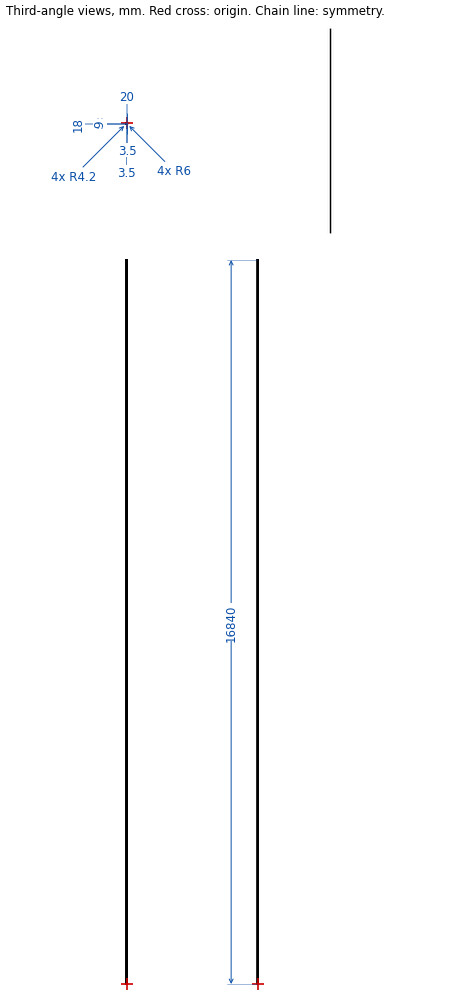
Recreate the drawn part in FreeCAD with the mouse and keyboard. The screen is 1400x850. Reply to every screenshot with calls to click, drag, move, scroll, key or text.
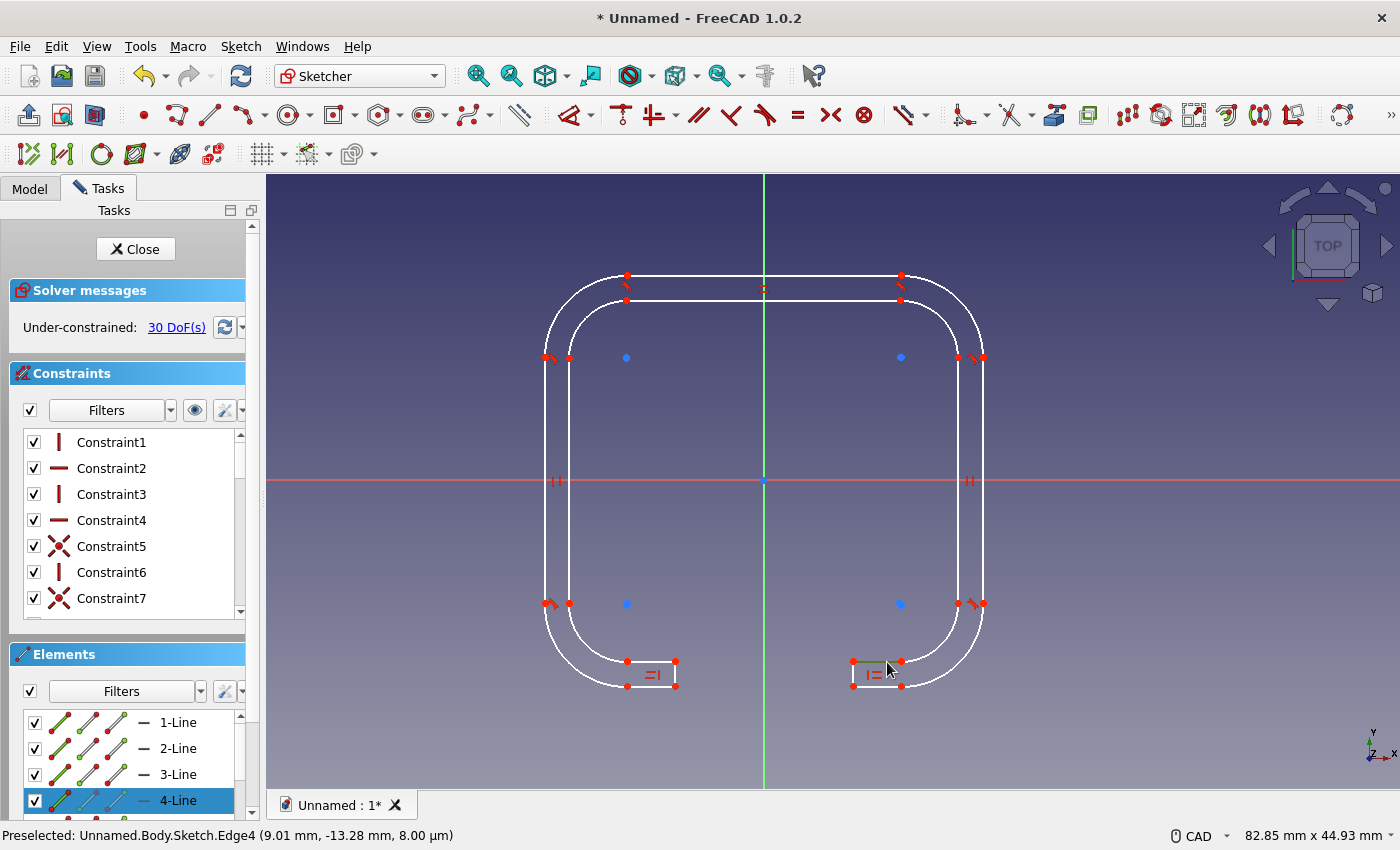
click(927, 655)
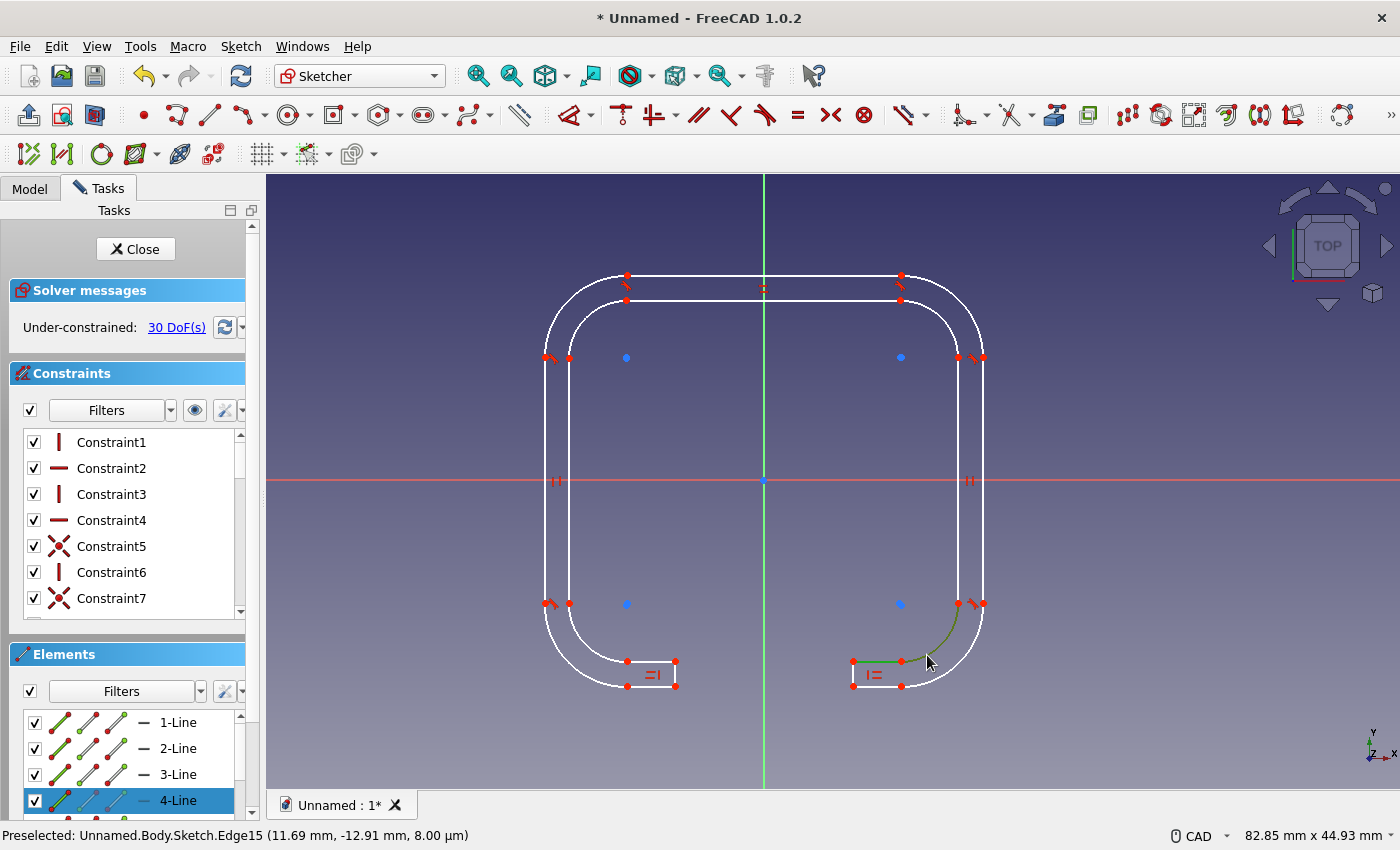
click(765, 116)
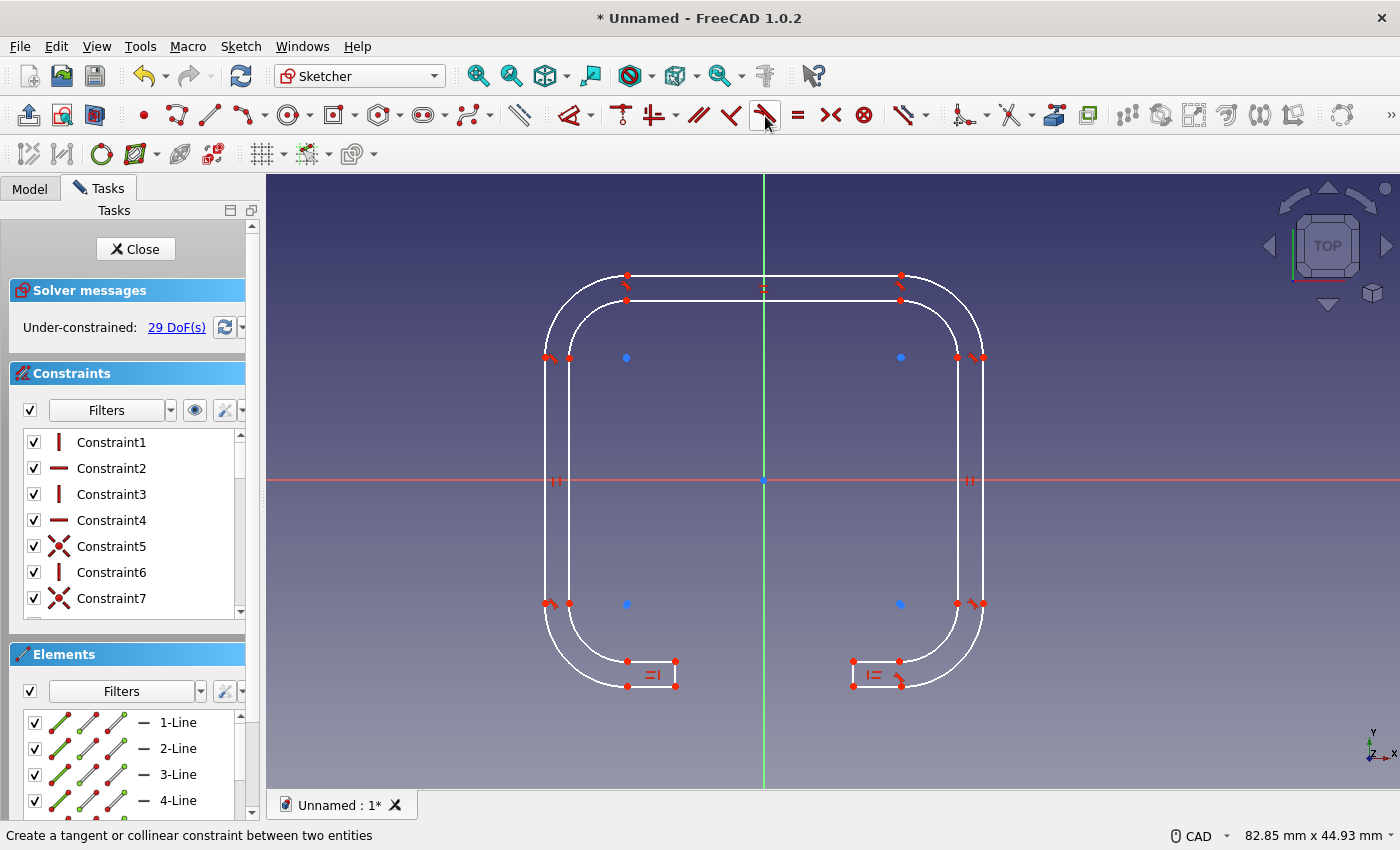
click(867, 687)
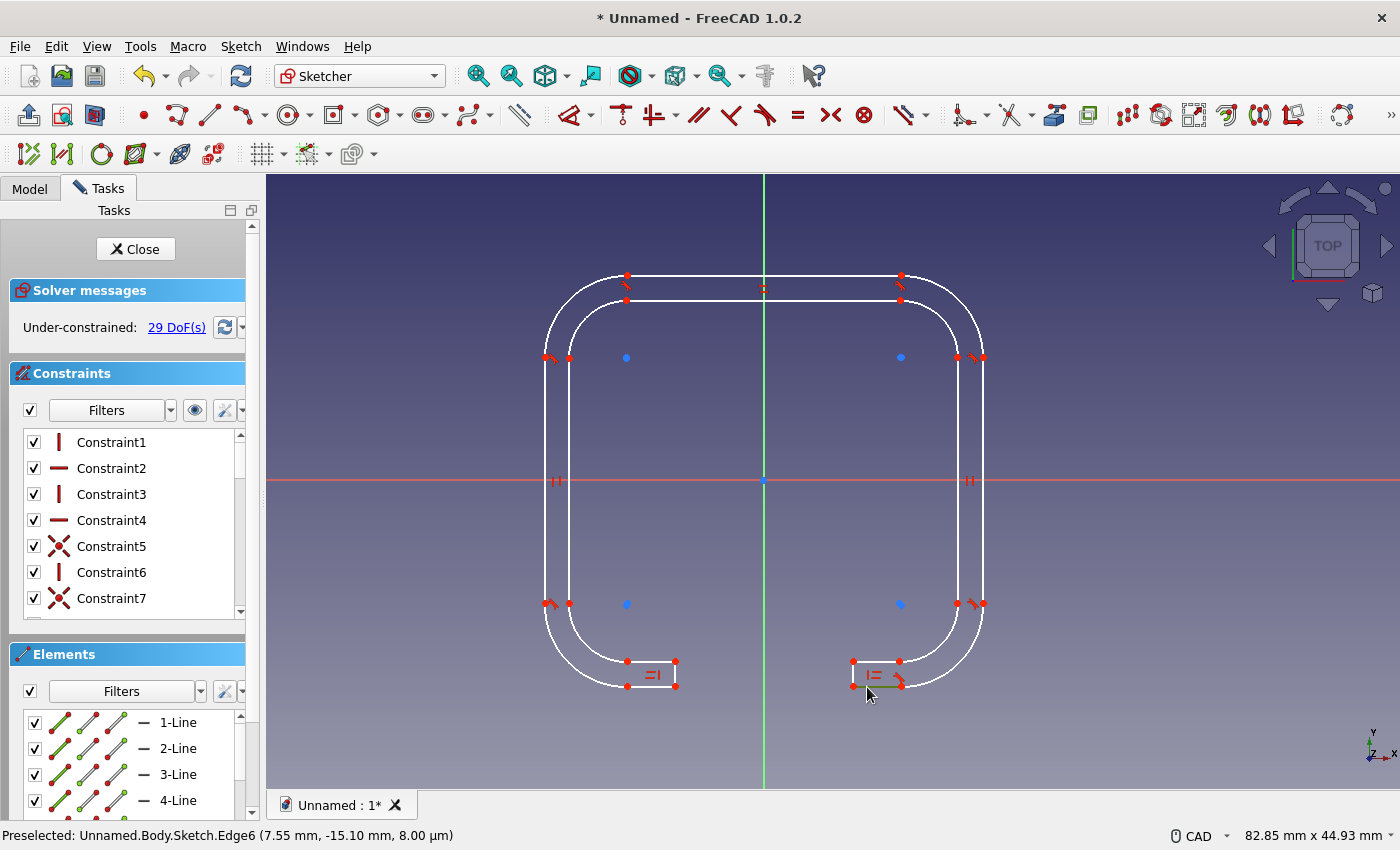
click(939, 678)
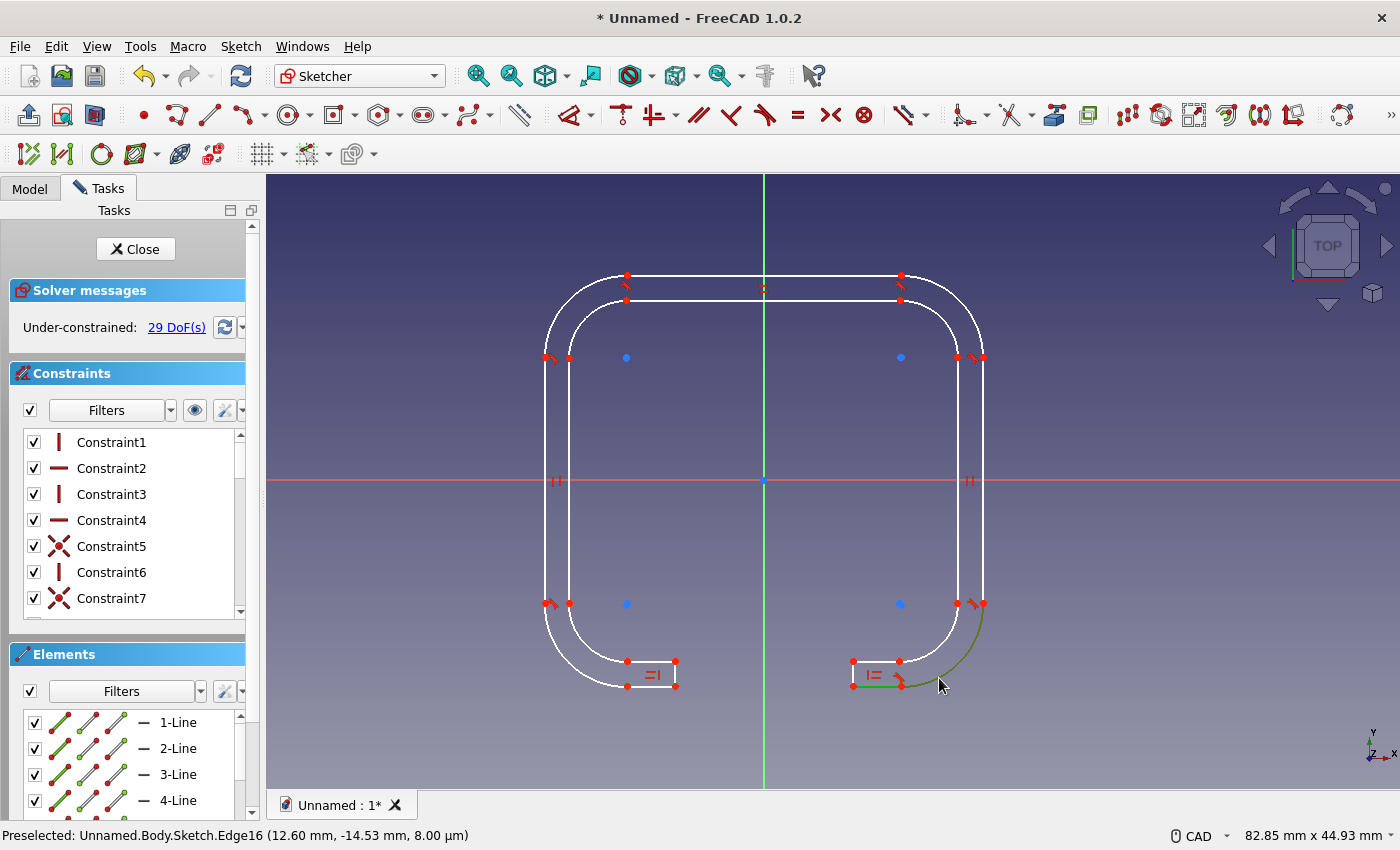
click(765, 116)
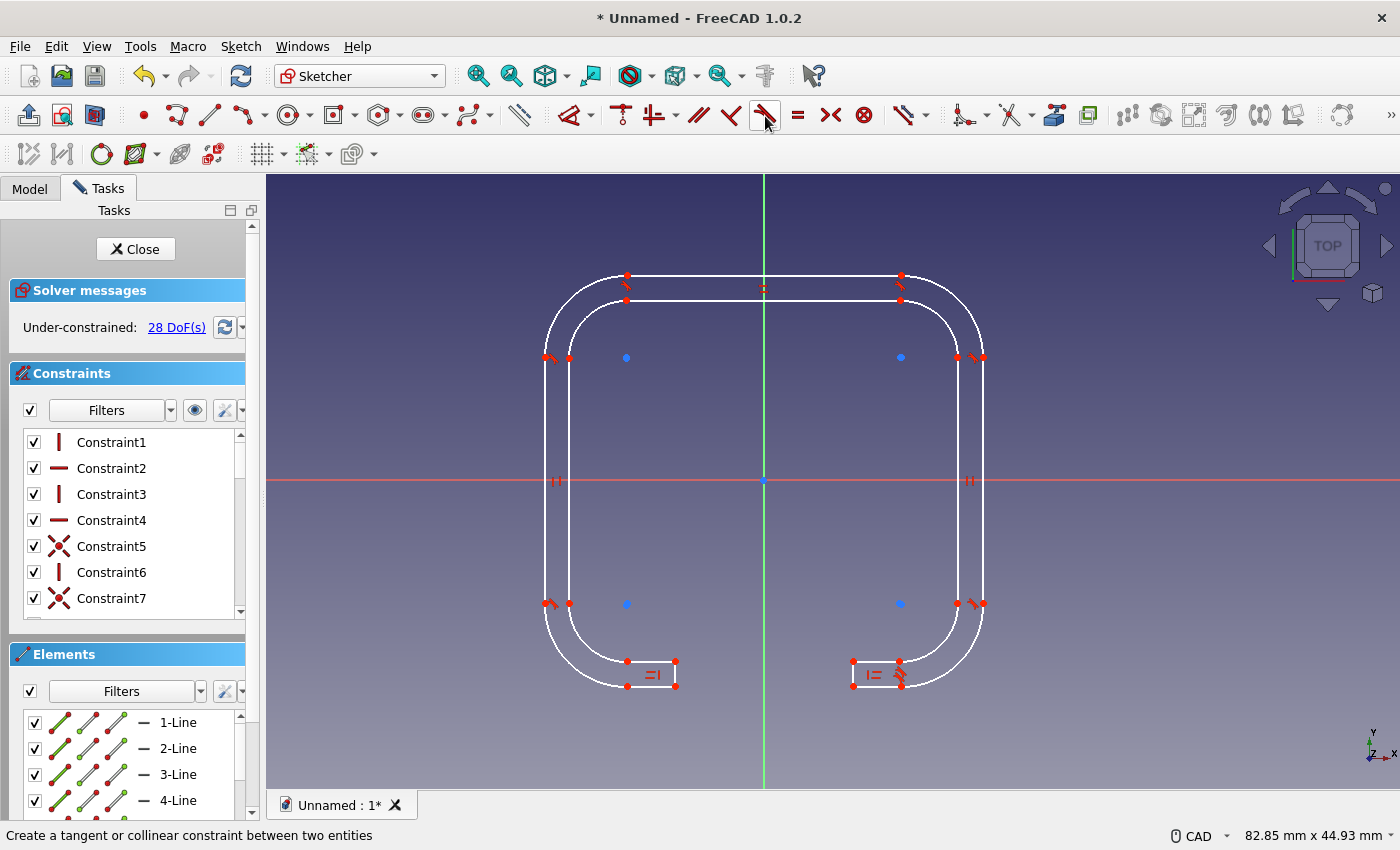
click(983, 530)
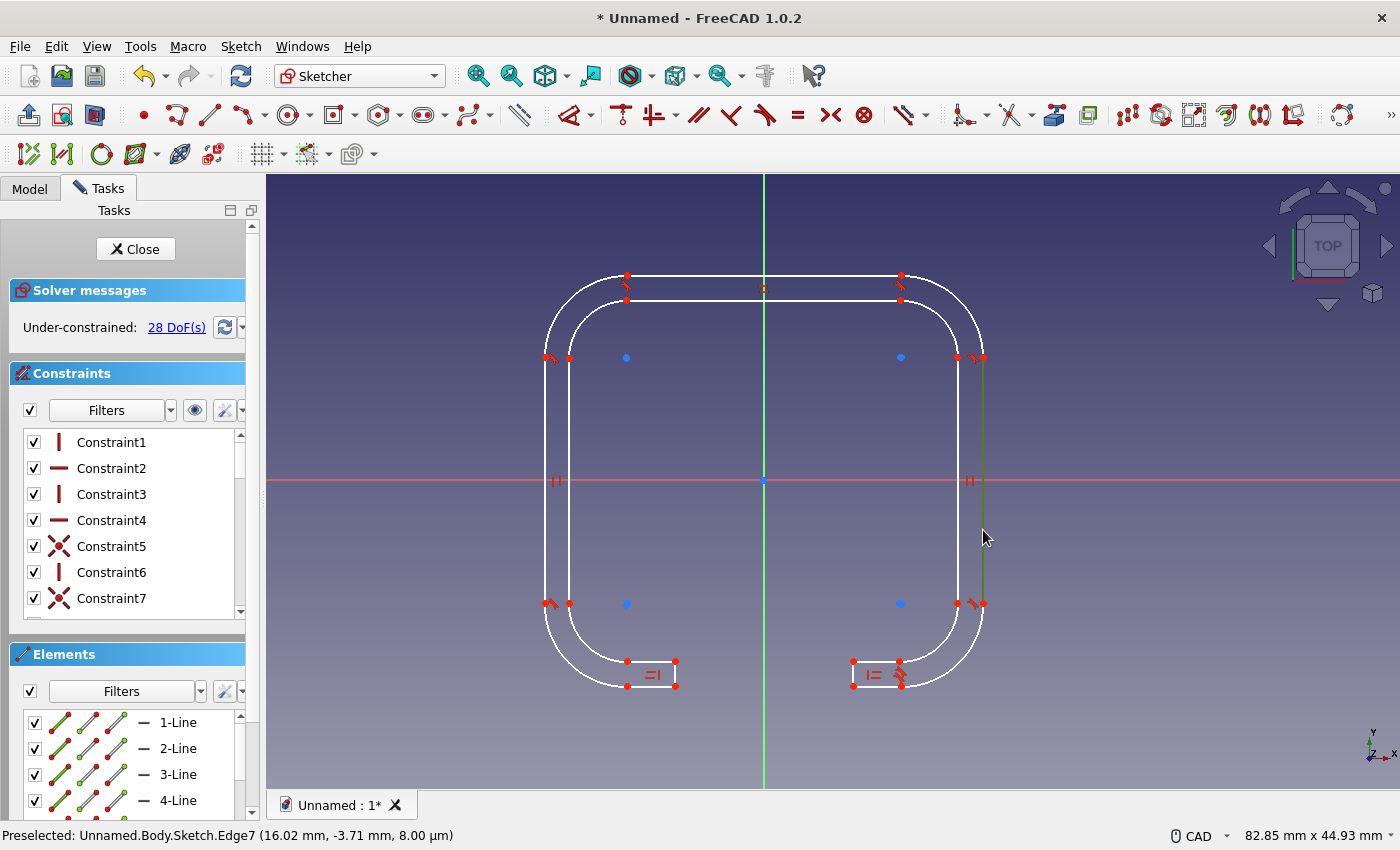
click(938, 678)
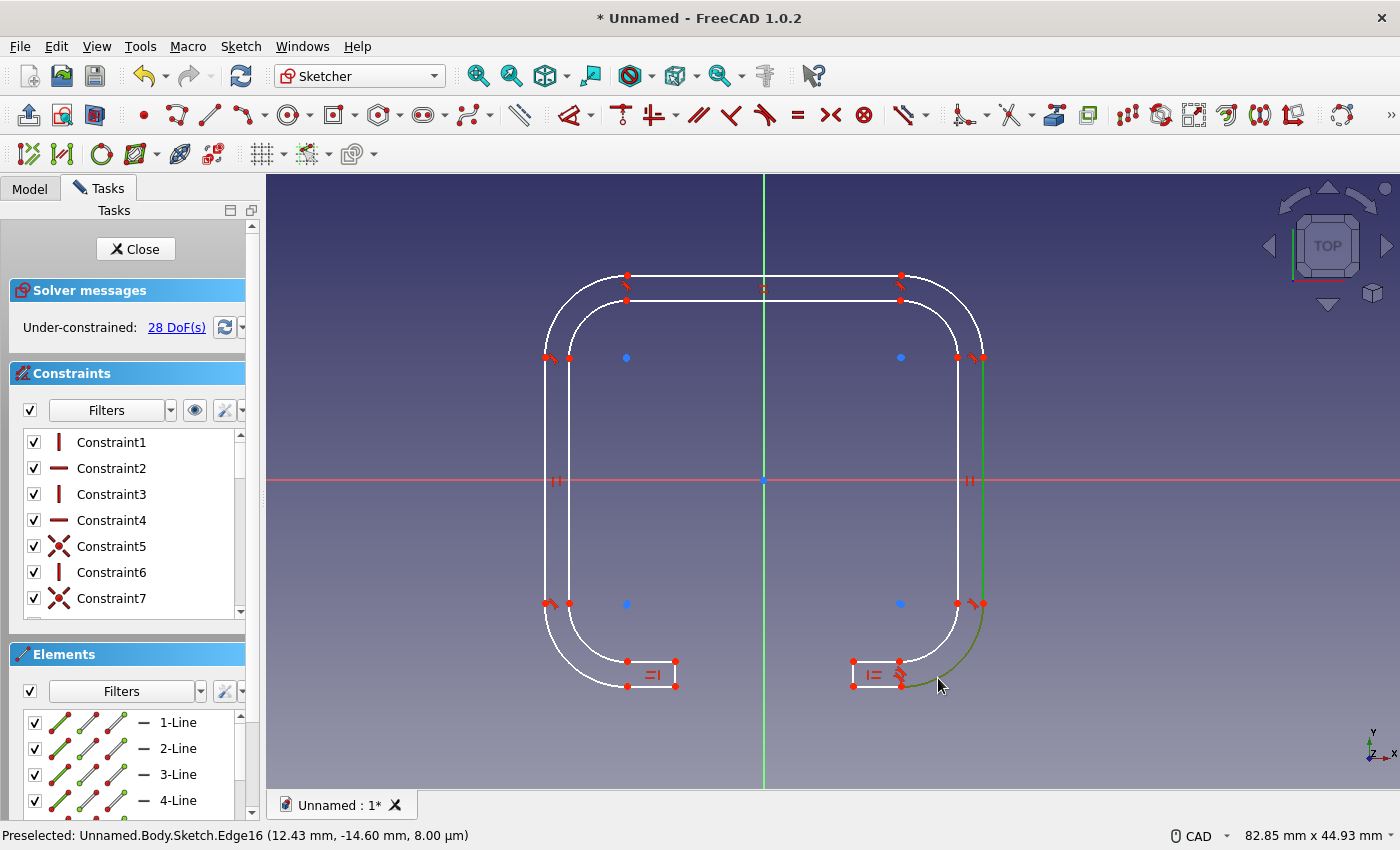
click(765, 116)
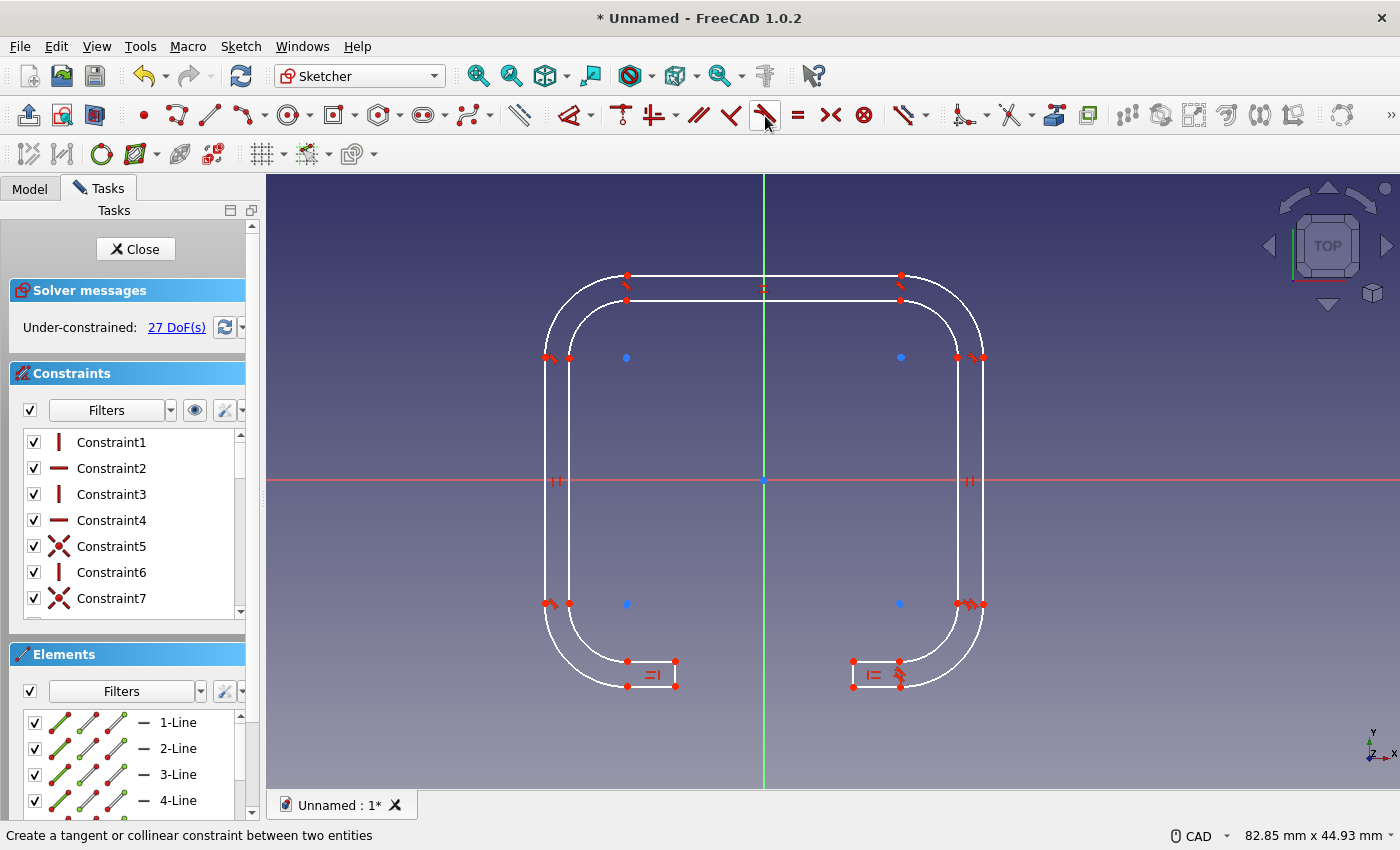
click(983, 530)